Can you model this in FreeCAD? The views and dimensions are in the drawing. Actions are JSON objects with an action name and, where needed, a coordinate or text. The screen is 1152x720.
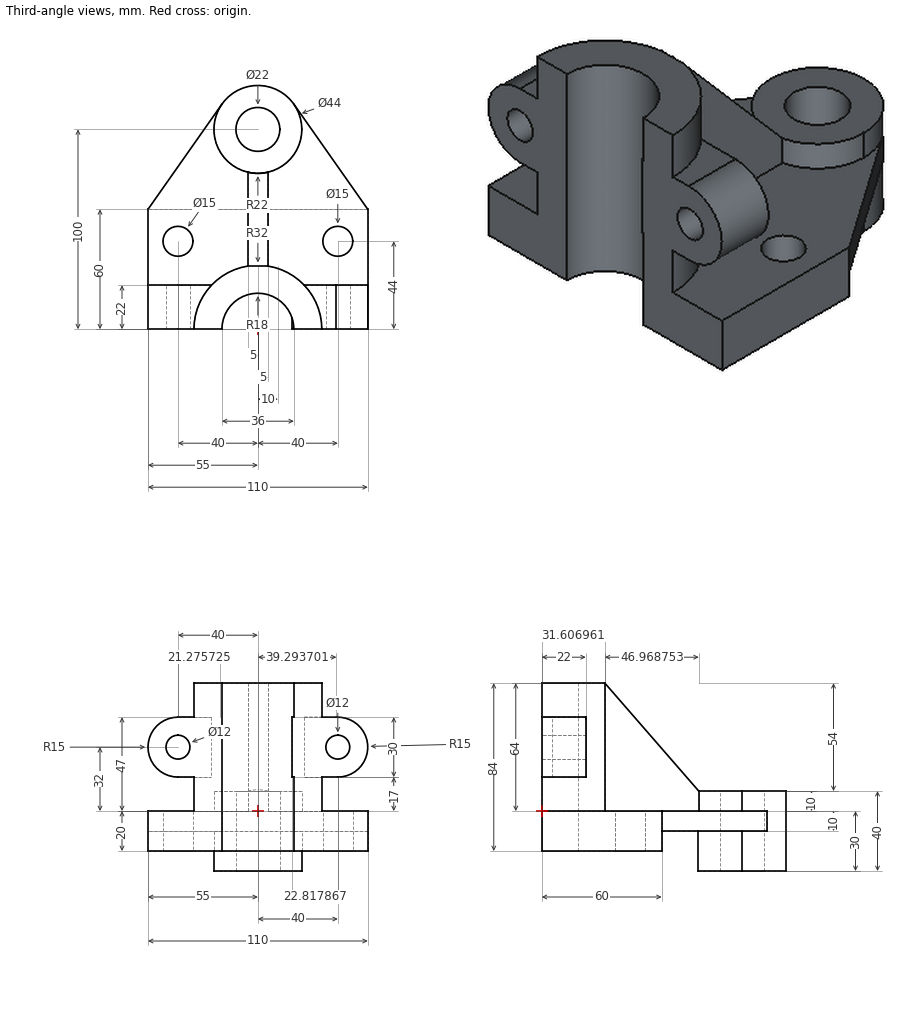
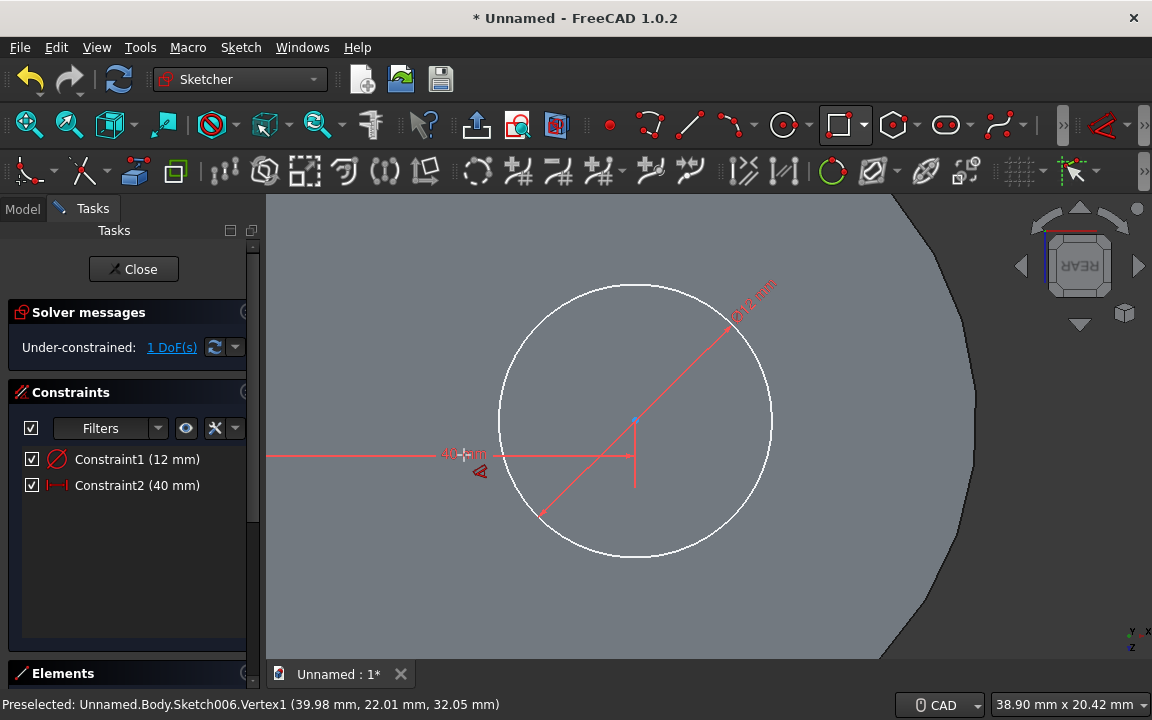
{"action": "left_click", "coordinate": [635, 421]}
{"action": "left_click", "coordinate": [669, 321]}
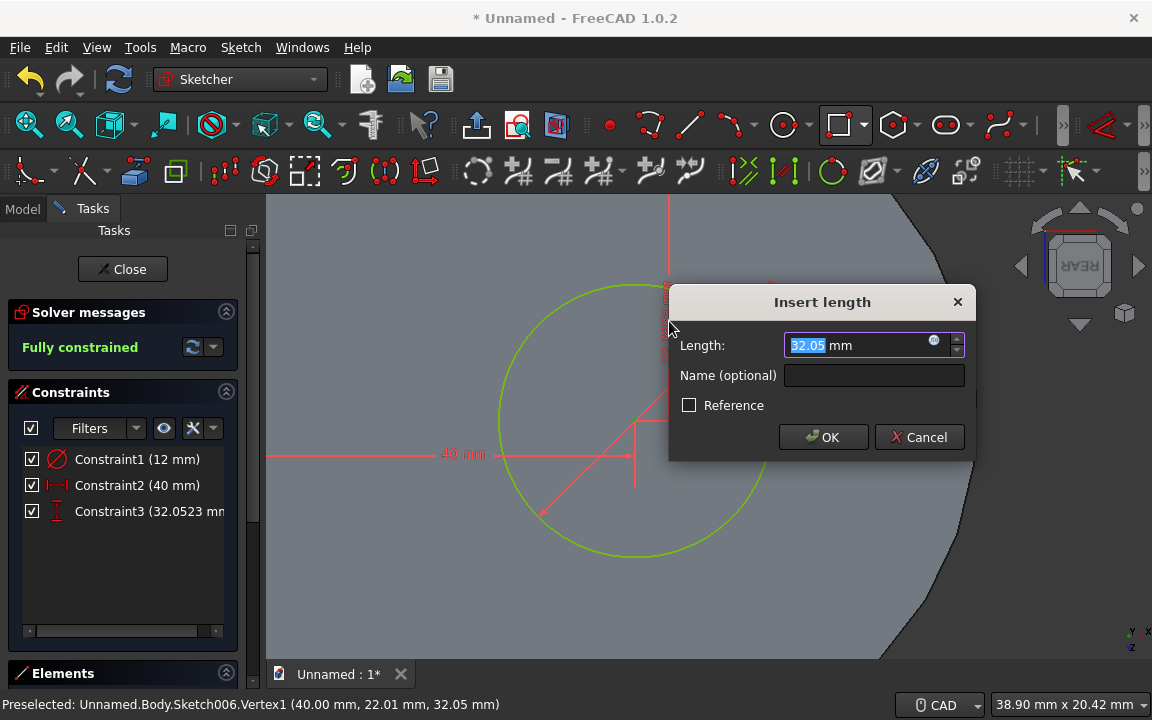
{"action": "type", "text": "32"}
{"action": "key", "text": "Return"}
{"action": "key", "text": "Escape"}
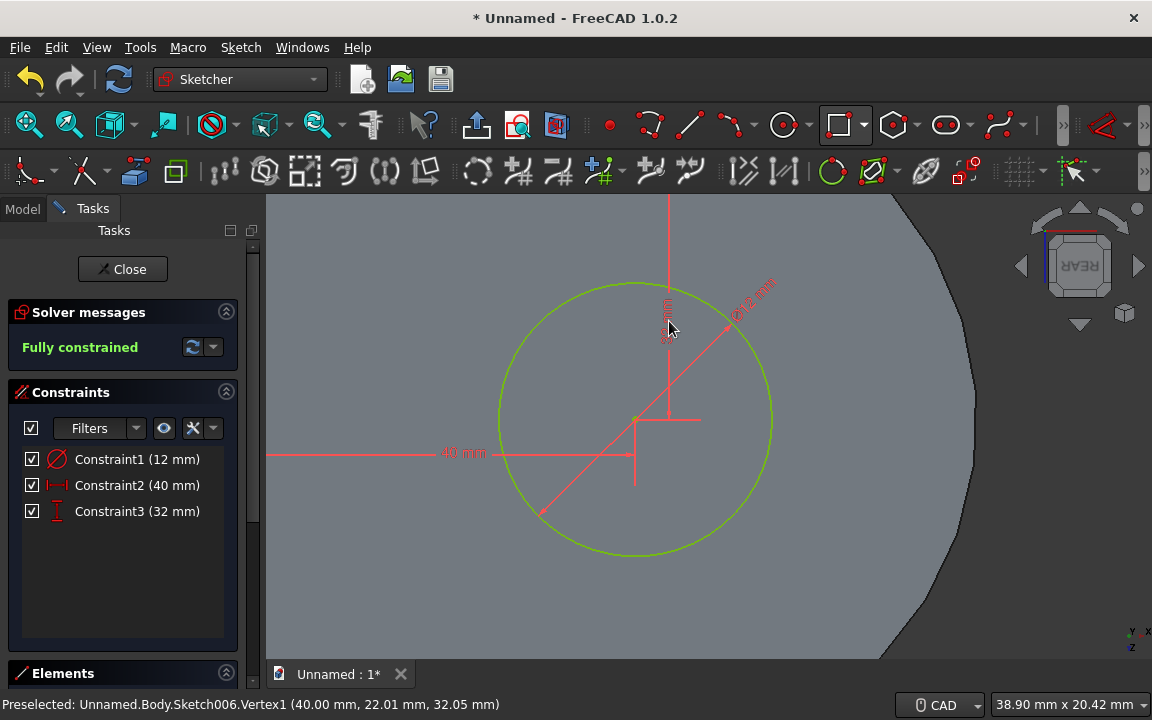
{"action": "left_click", "coordinate": [123, 269]}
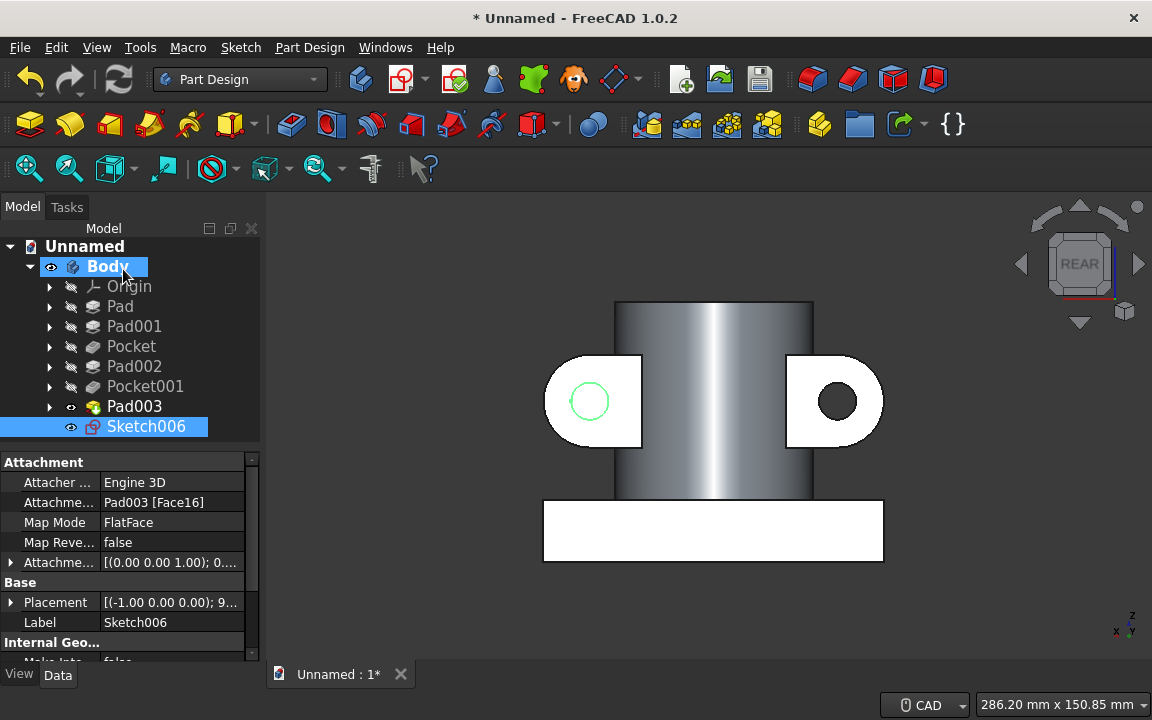
{"action": "left_click", "coordinate": [292, 124]}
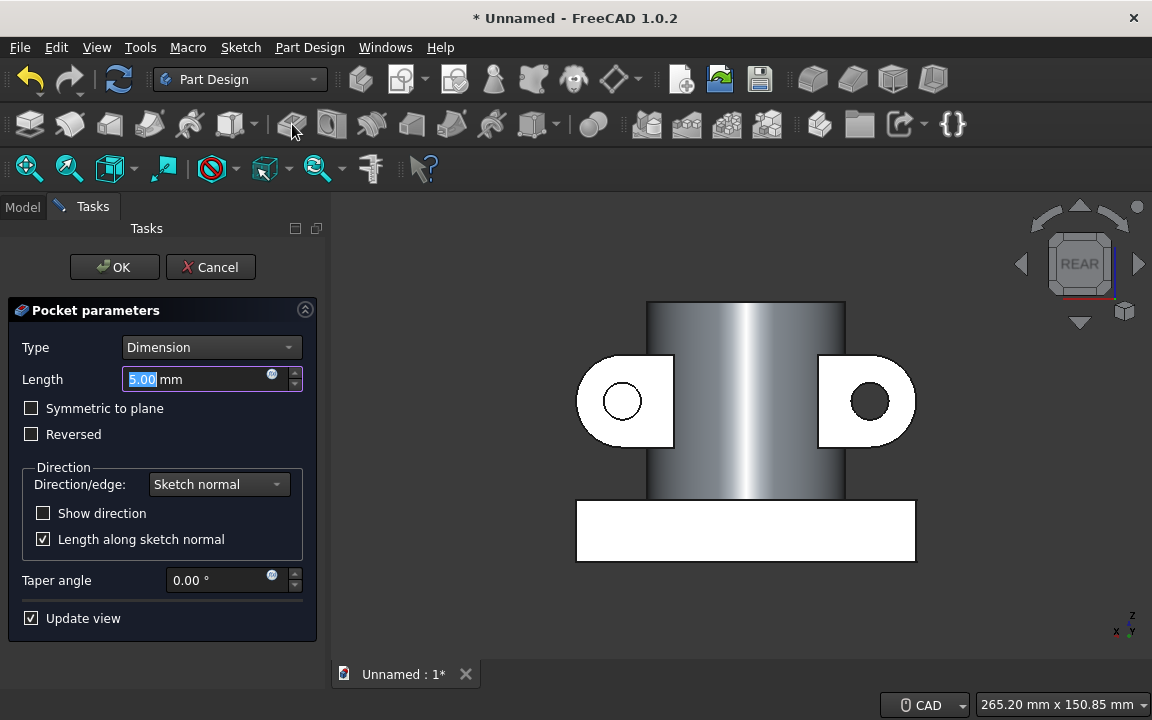
{"action": "type", "text": "22"}
{"action": "key", "text": "Tab"}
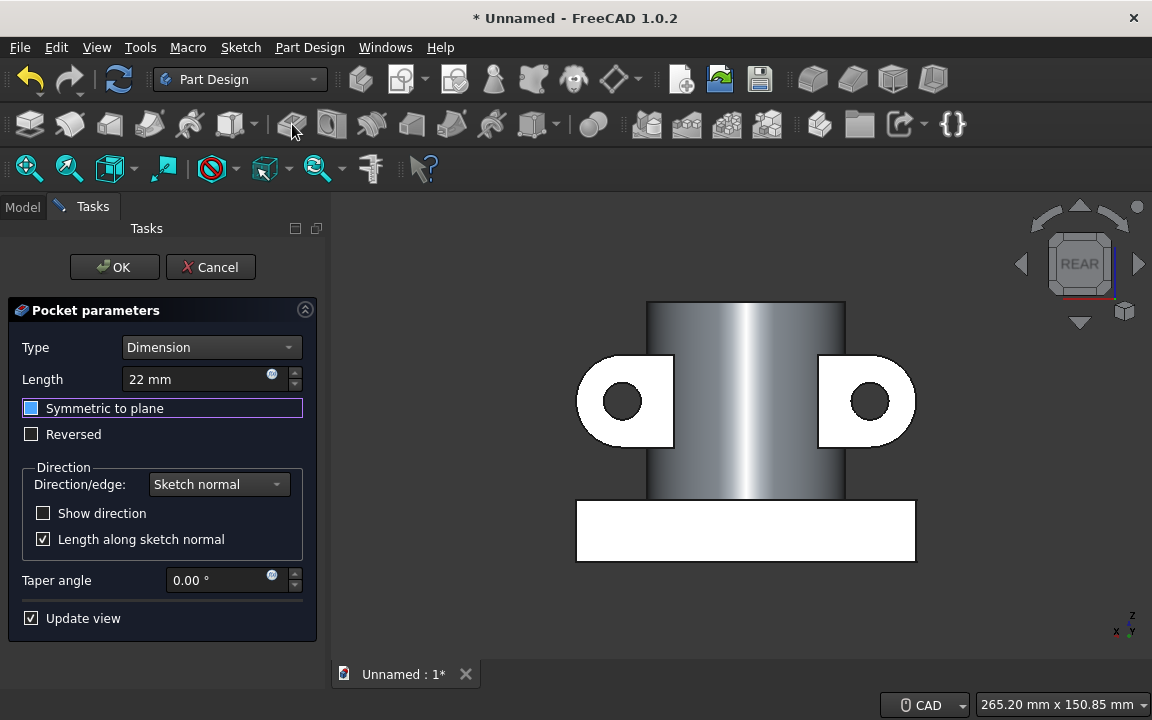
{"action": "left_click", "coordinate": [115, 267]}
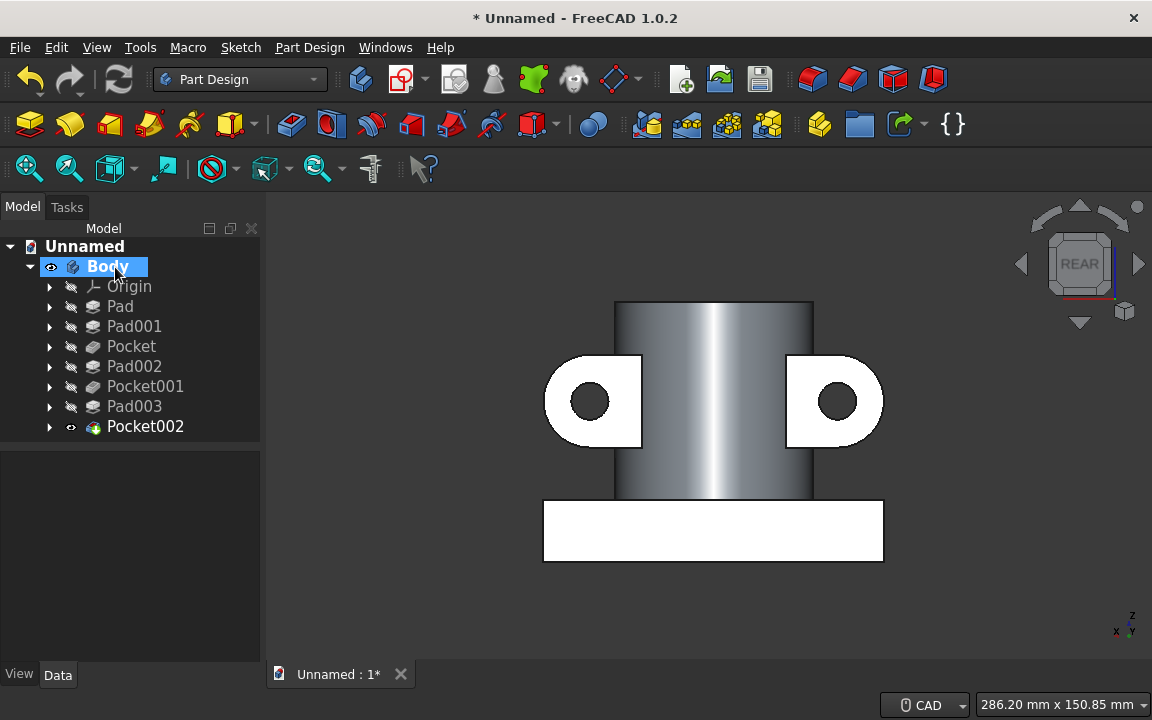
{"action": "left_click", "coordinate": [362, 80]}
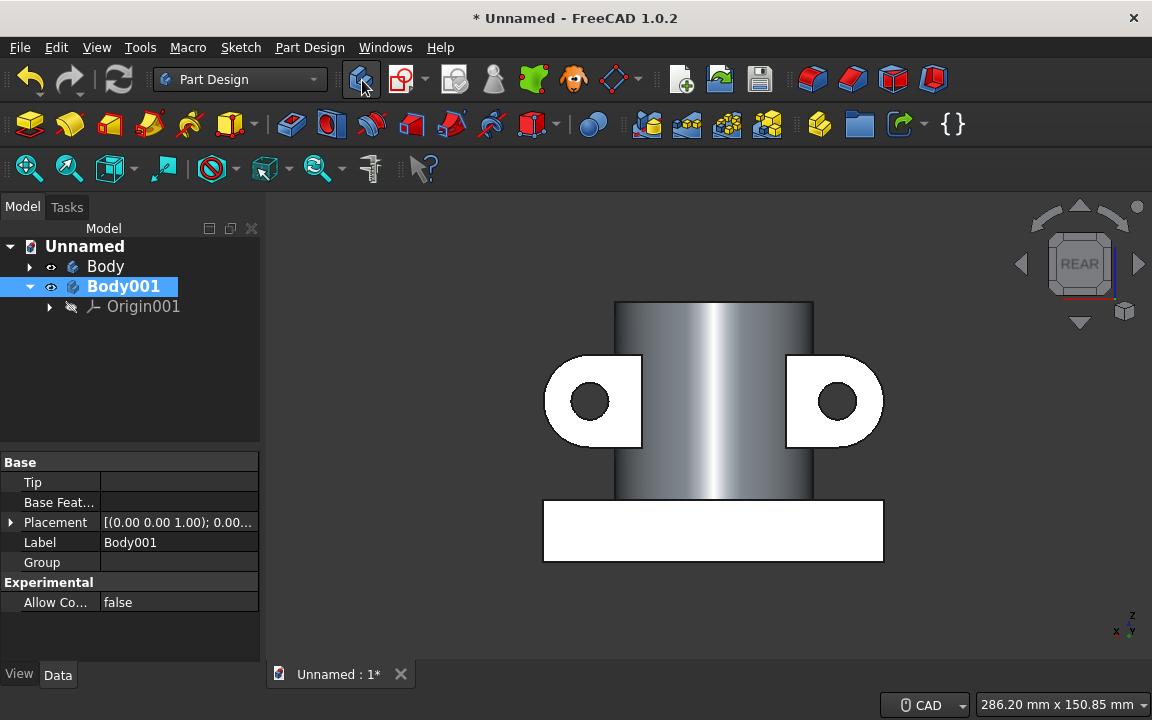
{"action": "left_click", "coordinate": [306, 619]}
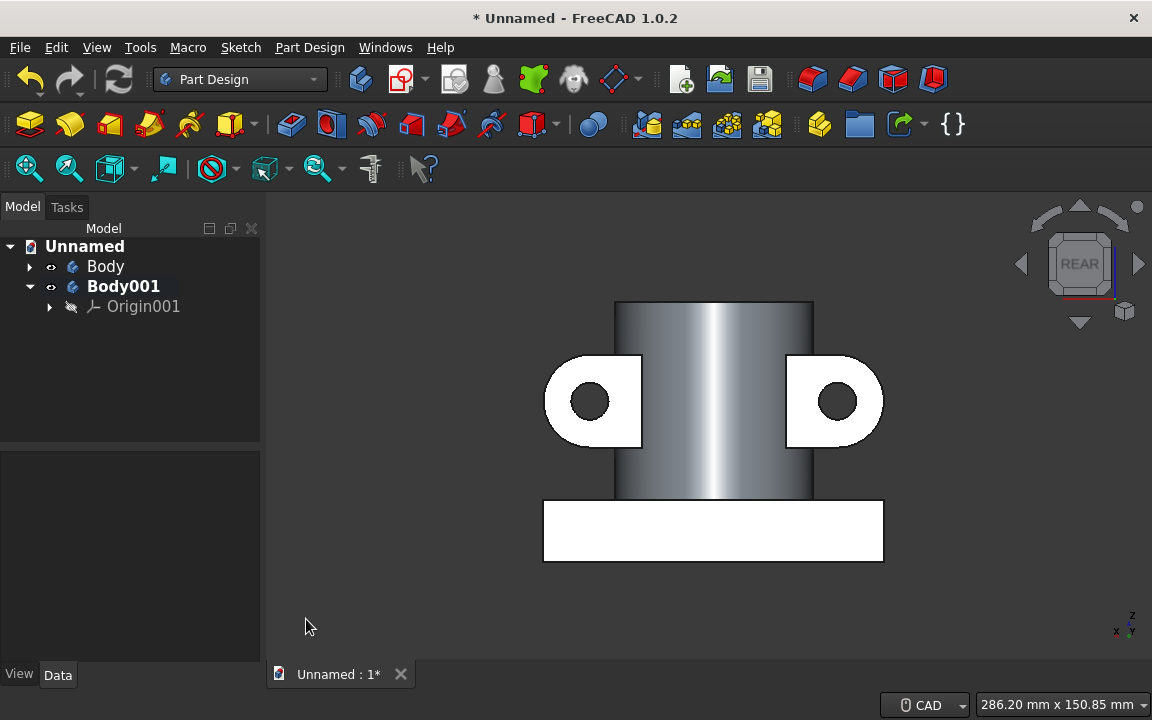
{"action": "left_click", "coordinate": [402, 80]}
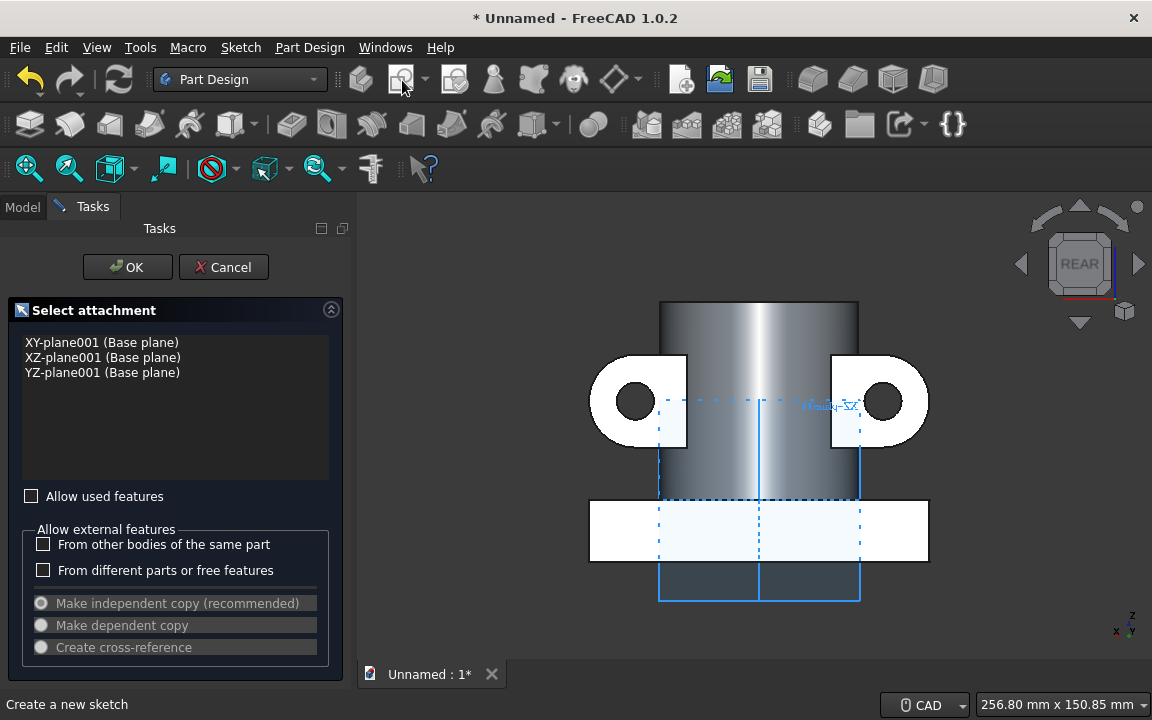
{"action": "left_click", "coordinate": [82, 342]}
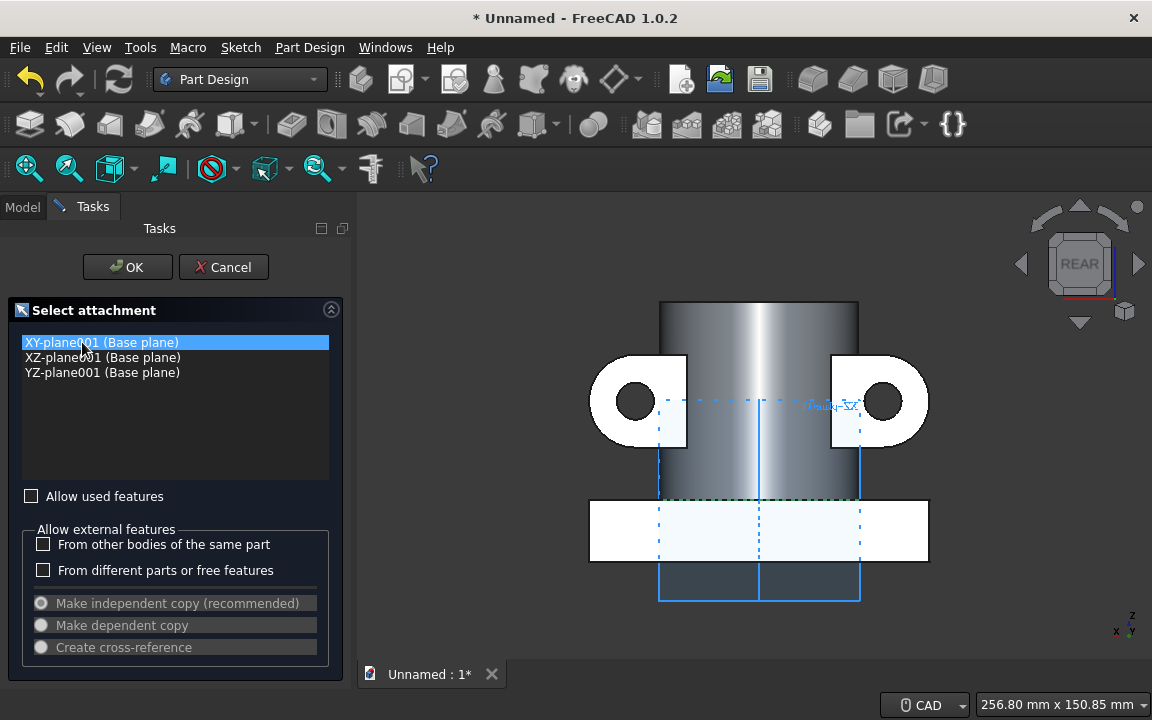
{"action": "left_click", "coordinate": [128, 267]}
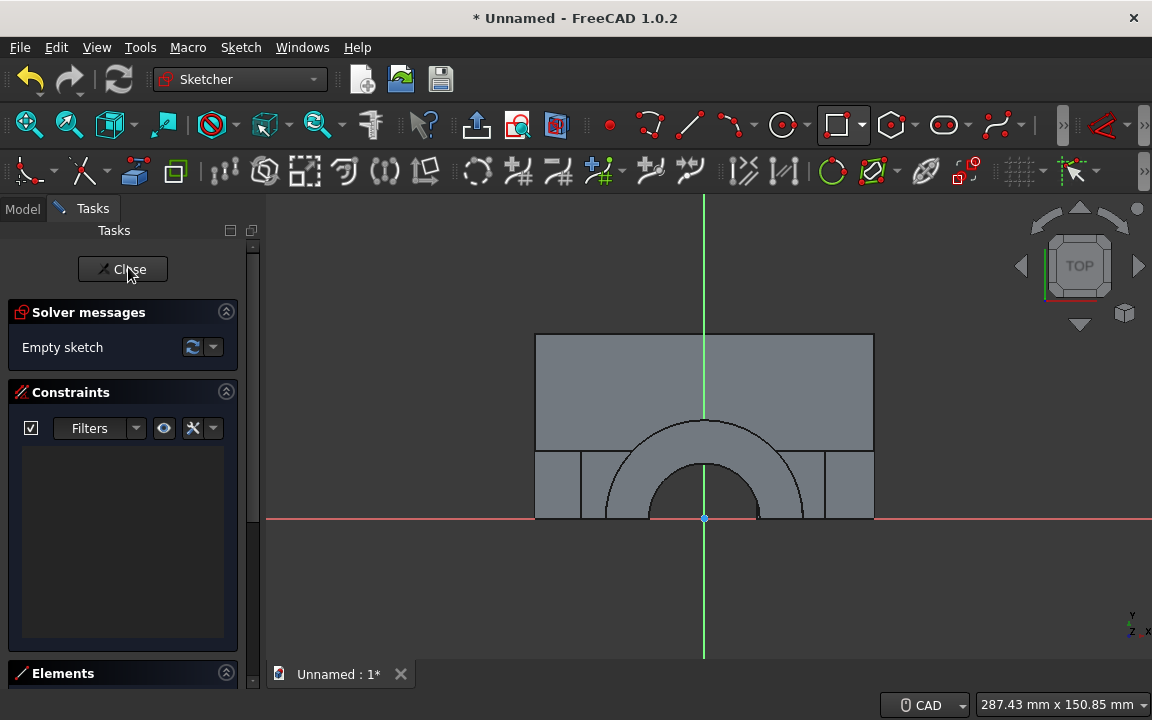
{"action": "scroll", "coordinate": [640, 426], "scroll_direction": "down", "scroll_amount": 5}